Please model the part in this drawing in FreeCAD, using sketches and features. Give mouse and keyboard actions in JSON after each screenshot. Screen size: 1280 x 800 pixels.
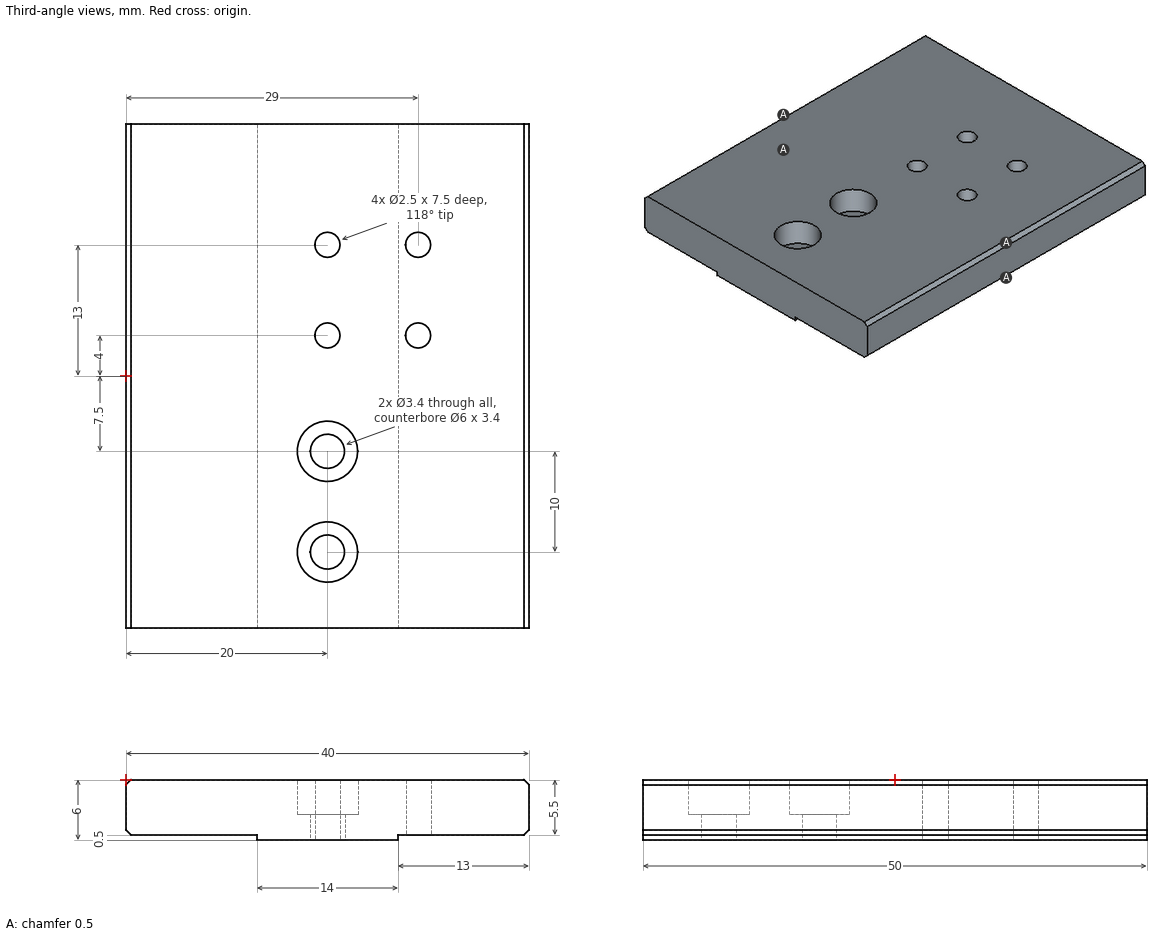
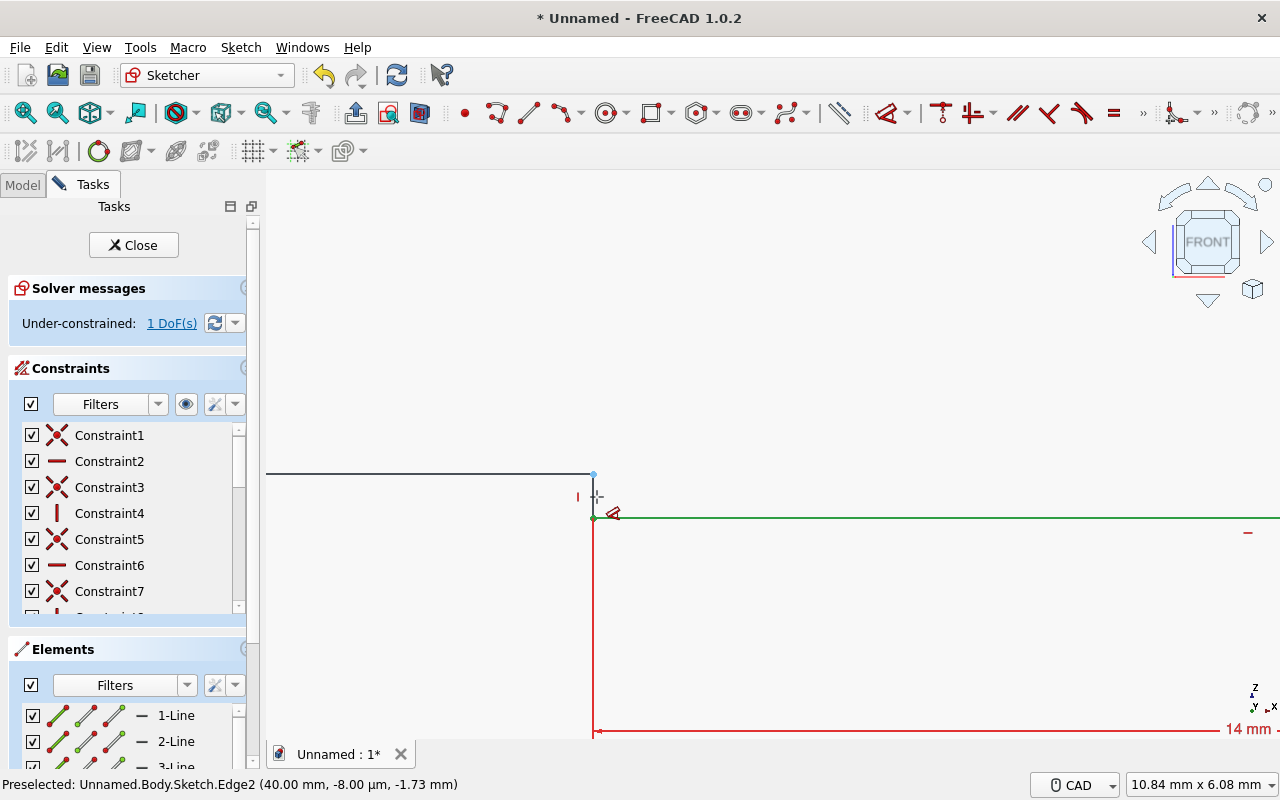
{"action": "left_click", "coordinate": [593, 496]}
{"action": "left_click", "coordinate": [559, 496]}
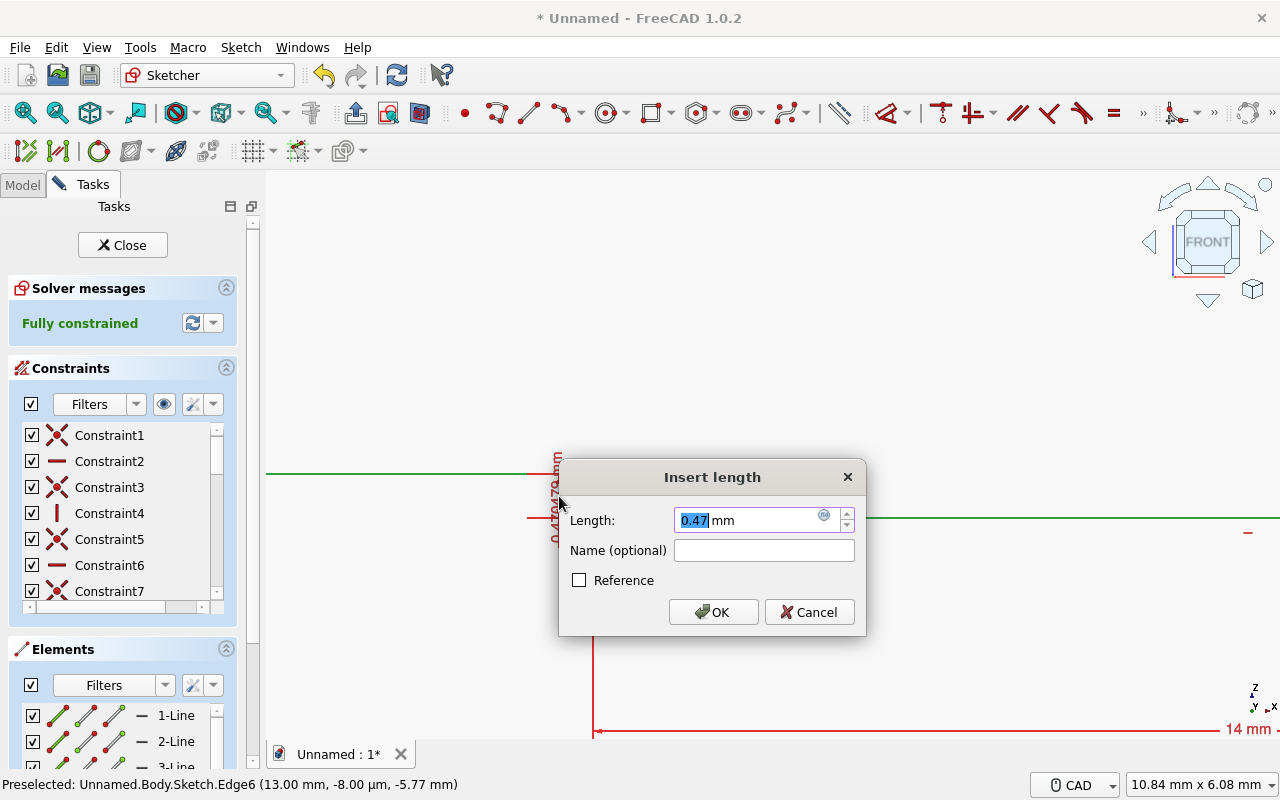
{"action": "type", "text": "0.5"}
{"action": "key", "text": "Return"}
{"action": "key", "text": "Escape"}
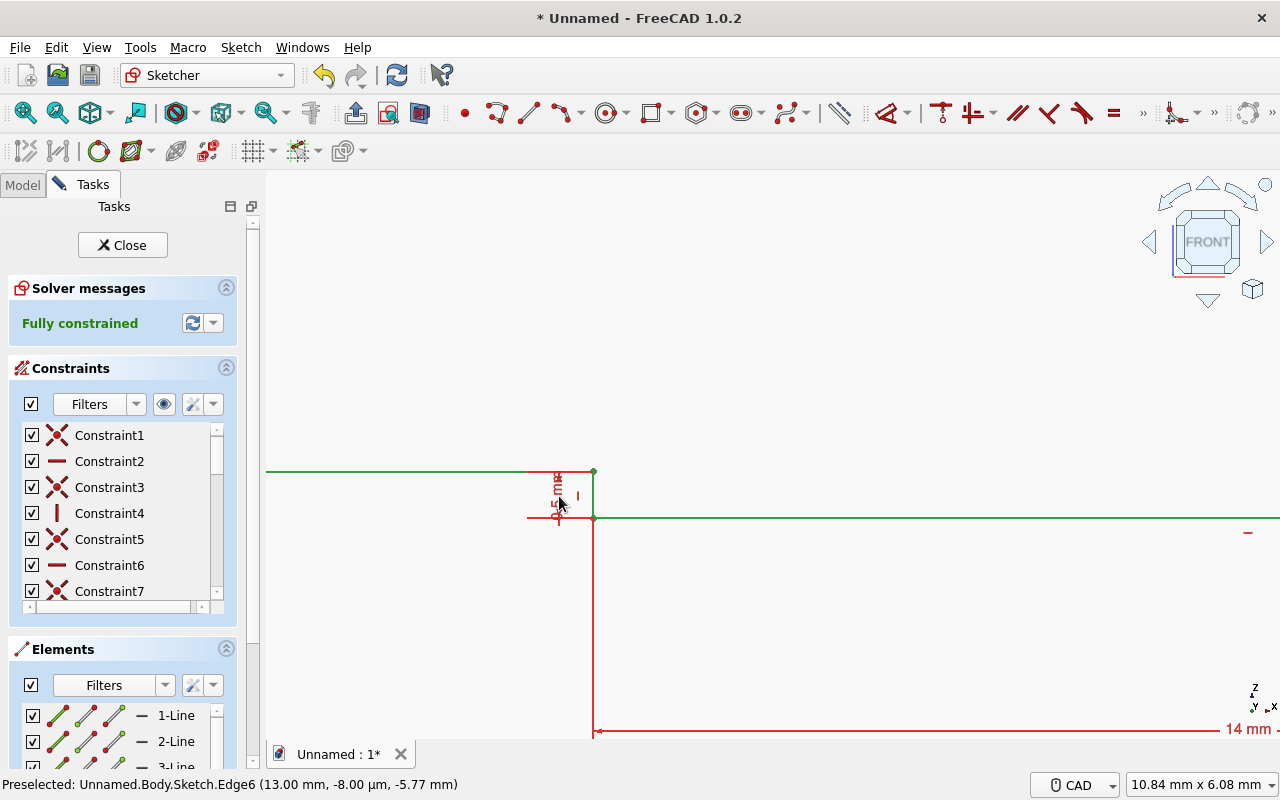
{"action": "left_click", "coordinate": [123, 245]}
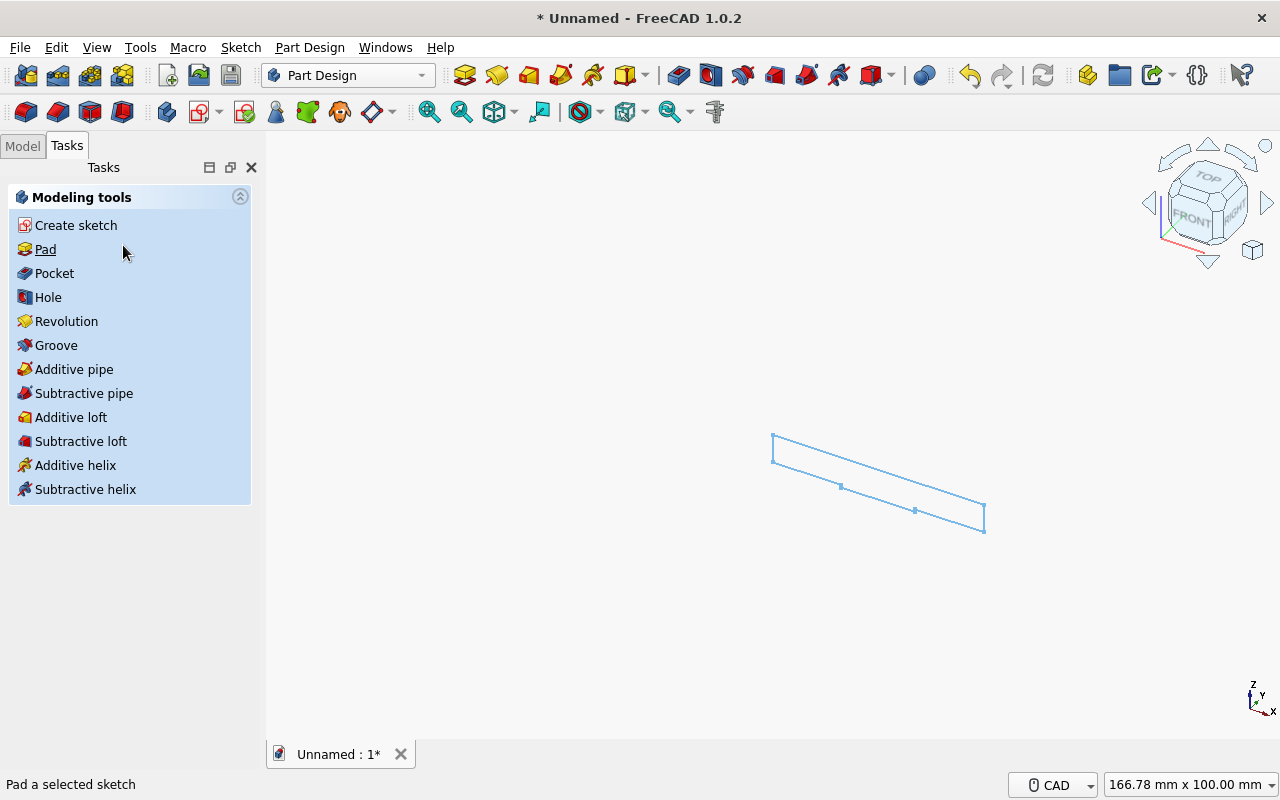
{"action": "left_click", "coordinate": [466, 76]}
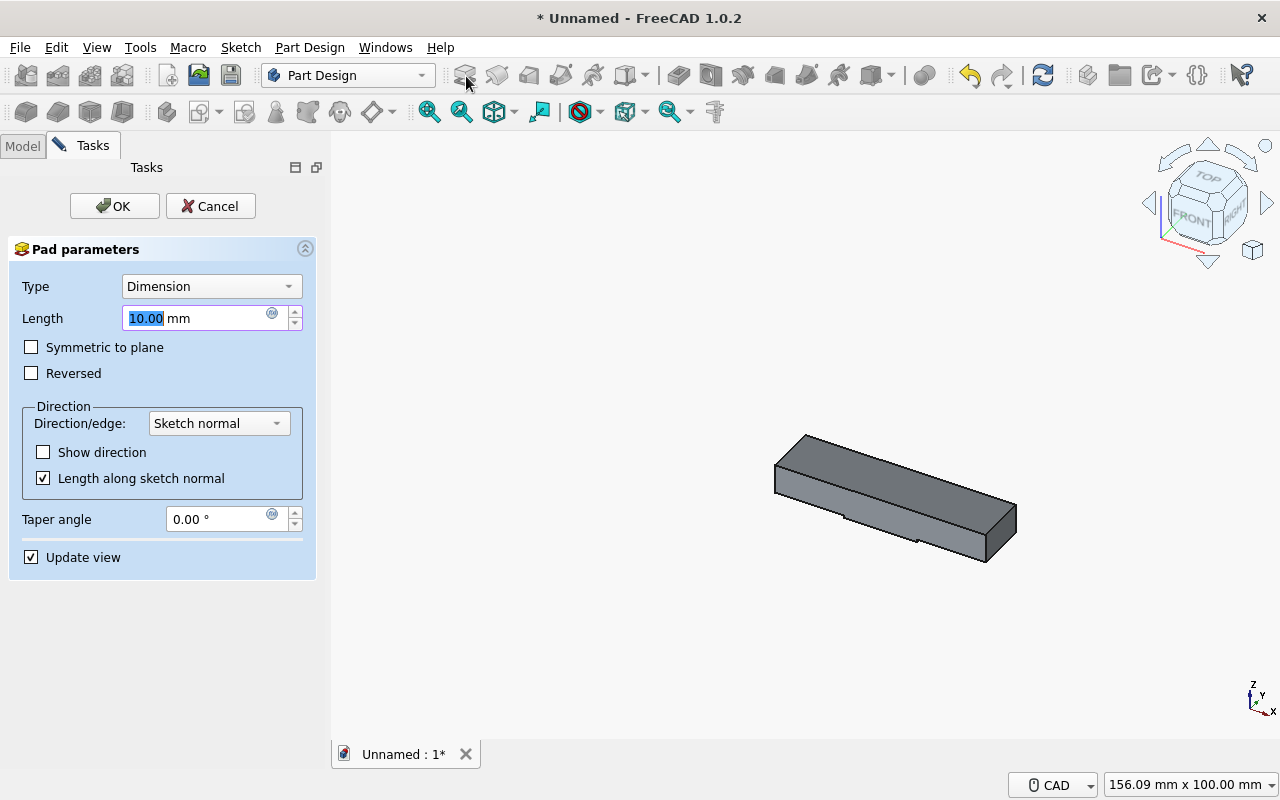
{"action": "type", "text": "50"}
{"action": "key", "text": "Tab"}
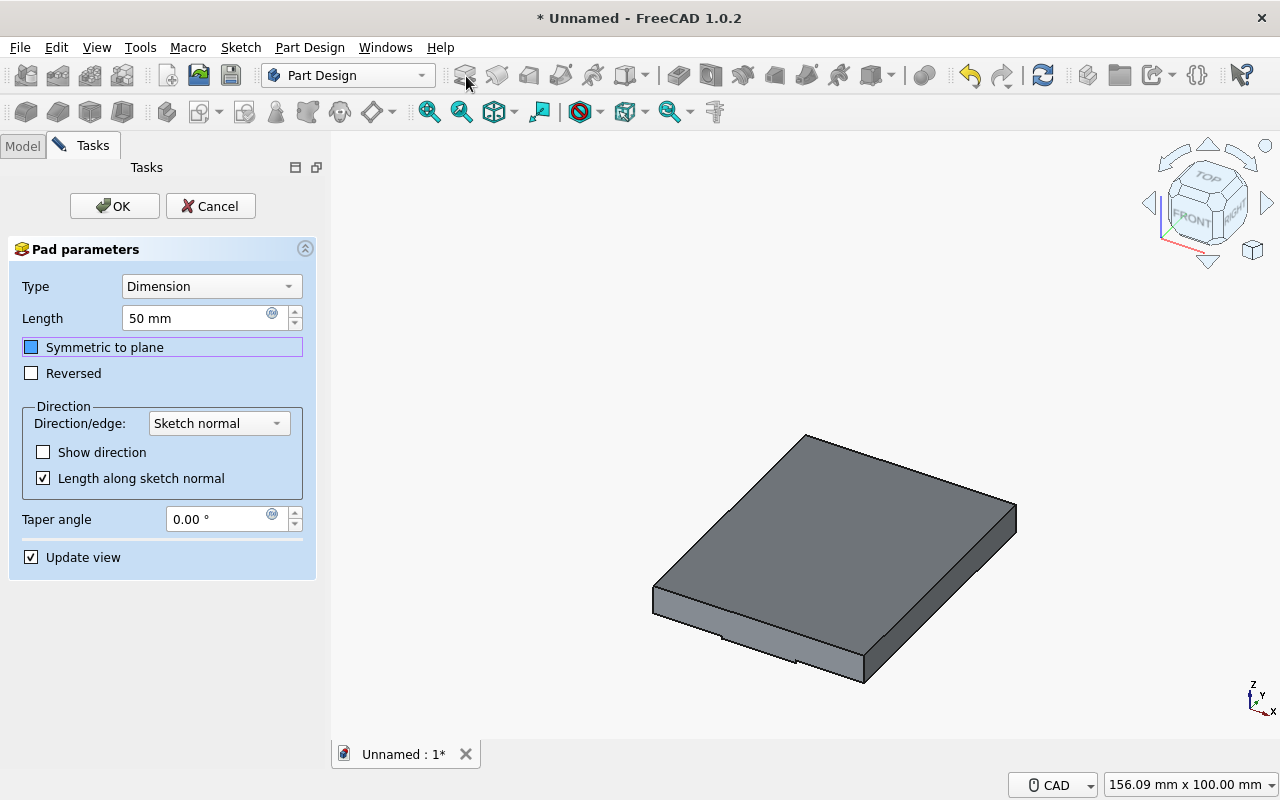
{"action": "left_click", "coordinate": [30, 347]}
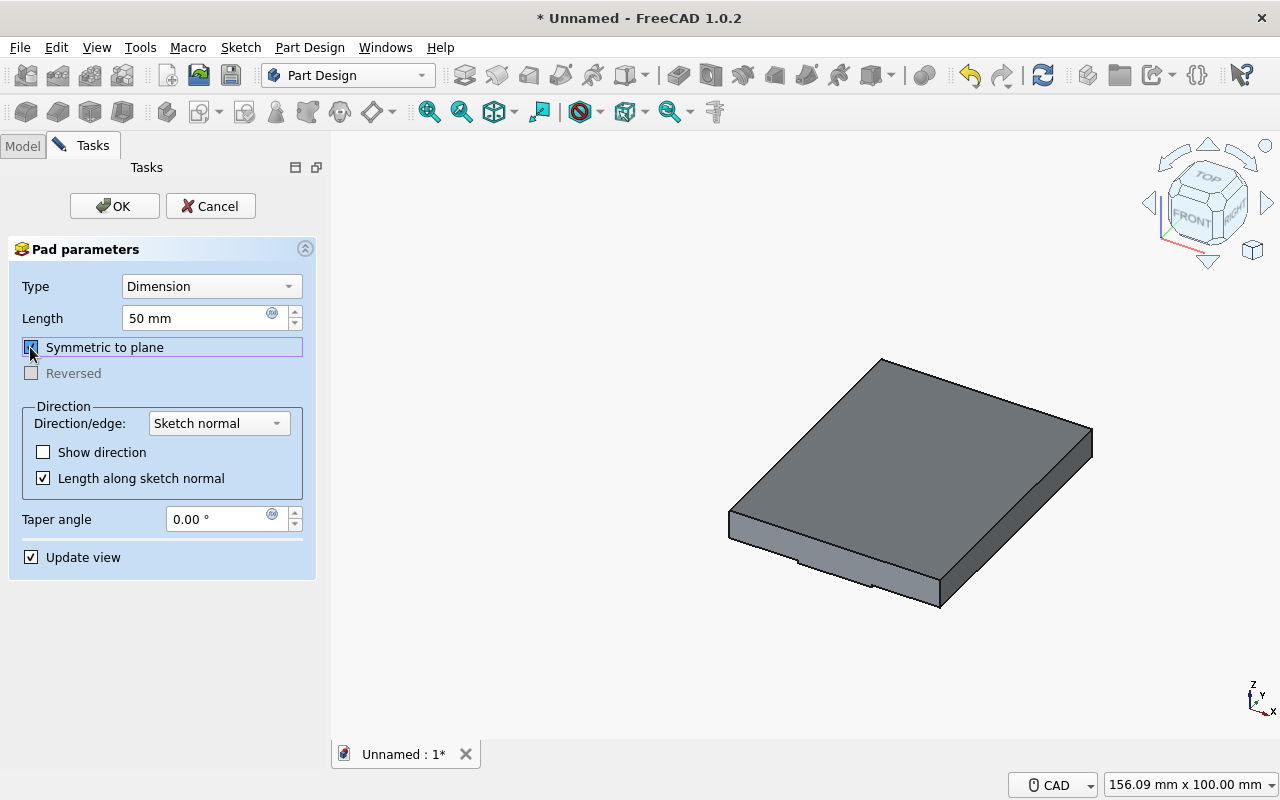
{"action": "left_click", "coordinate": [115, 206]}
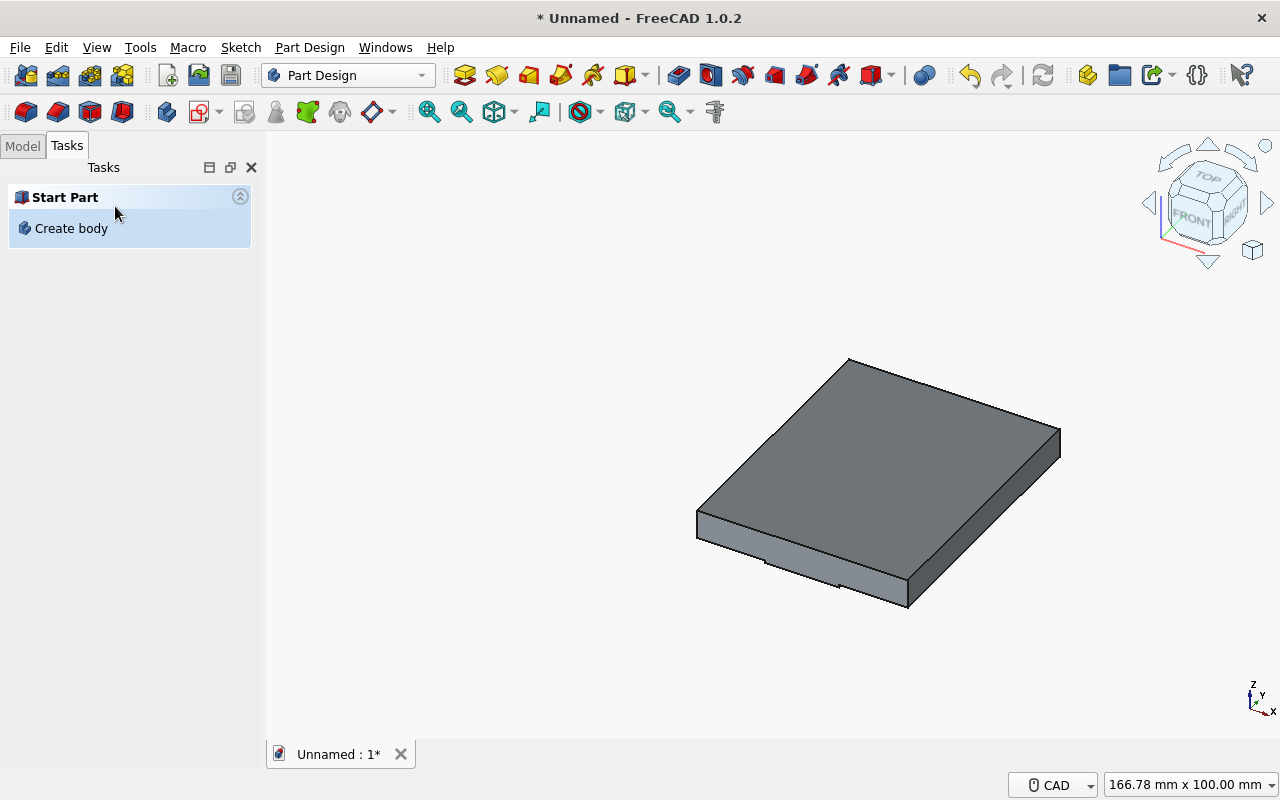
{"action": "left_click", "coordinate": [430, 112]}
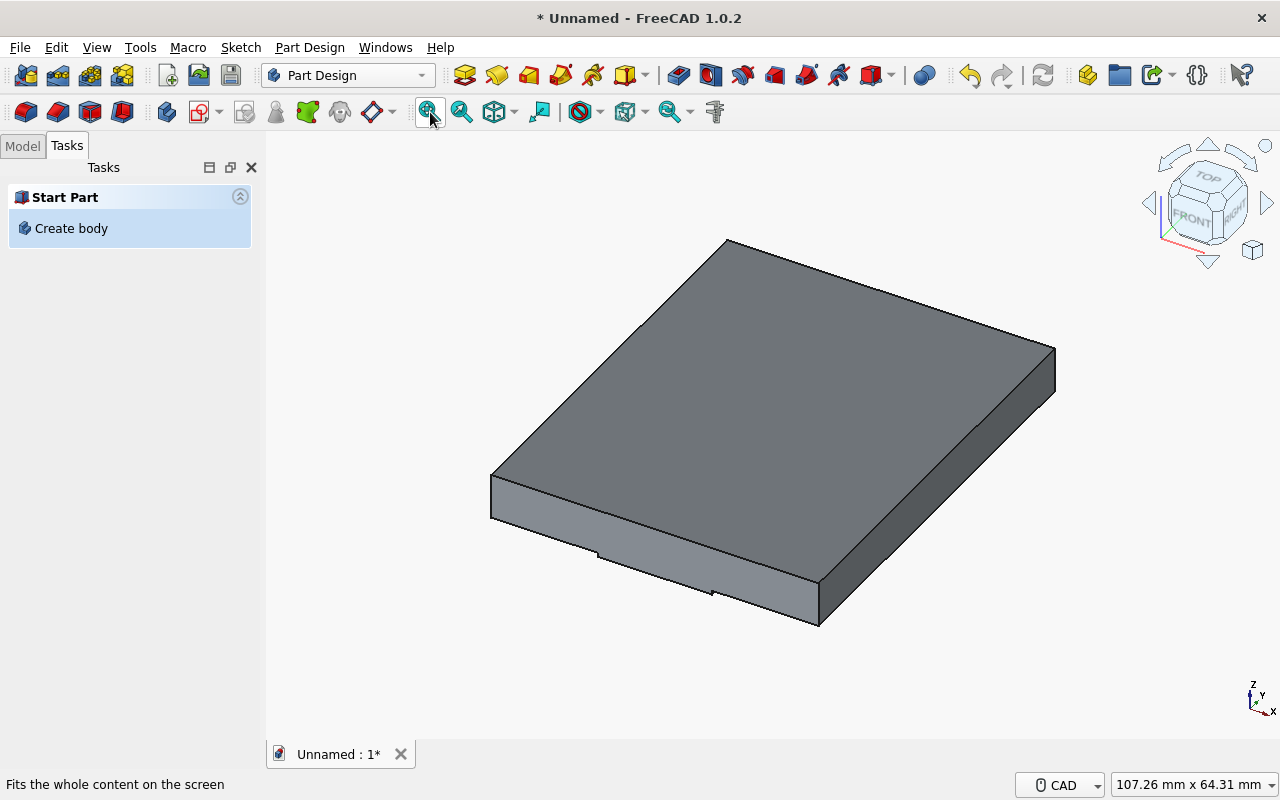
{"action": "left_click", "coordinate": [937, 465]}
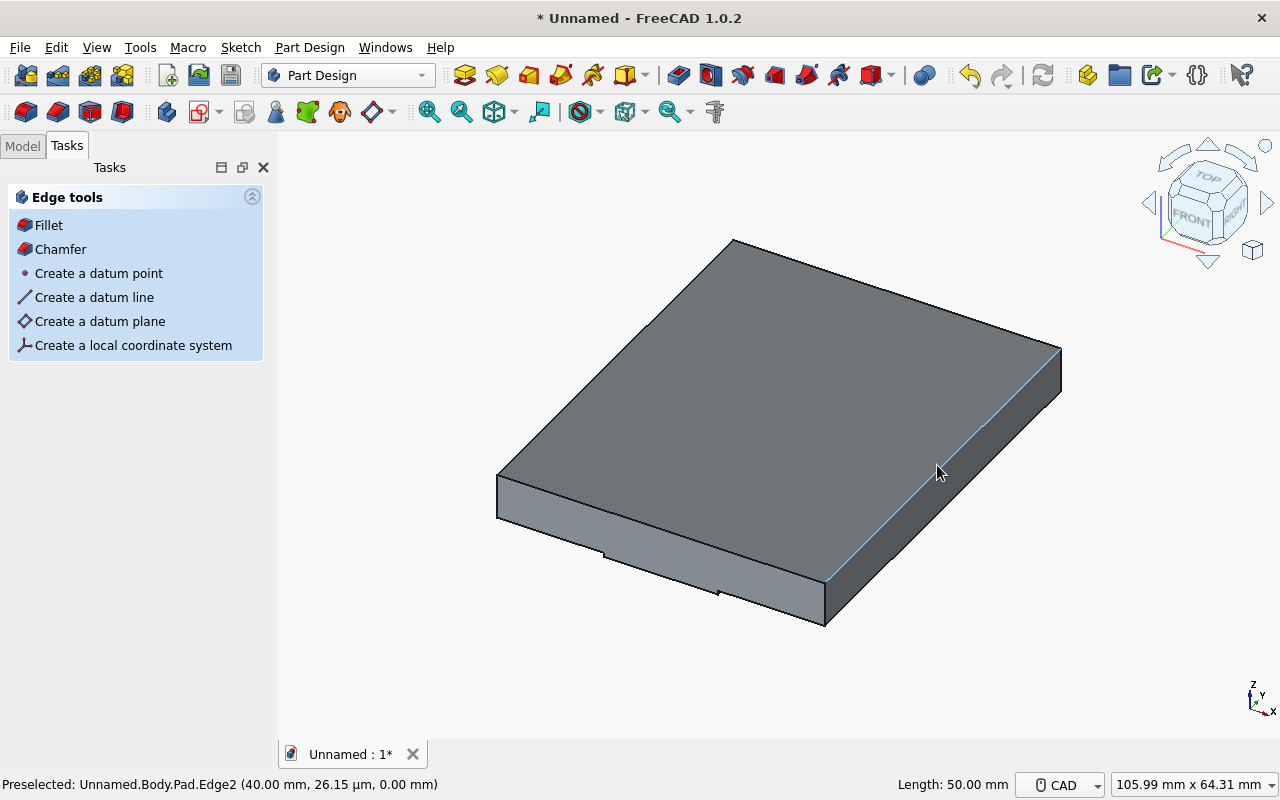
{"action": "key", "text": "0"}